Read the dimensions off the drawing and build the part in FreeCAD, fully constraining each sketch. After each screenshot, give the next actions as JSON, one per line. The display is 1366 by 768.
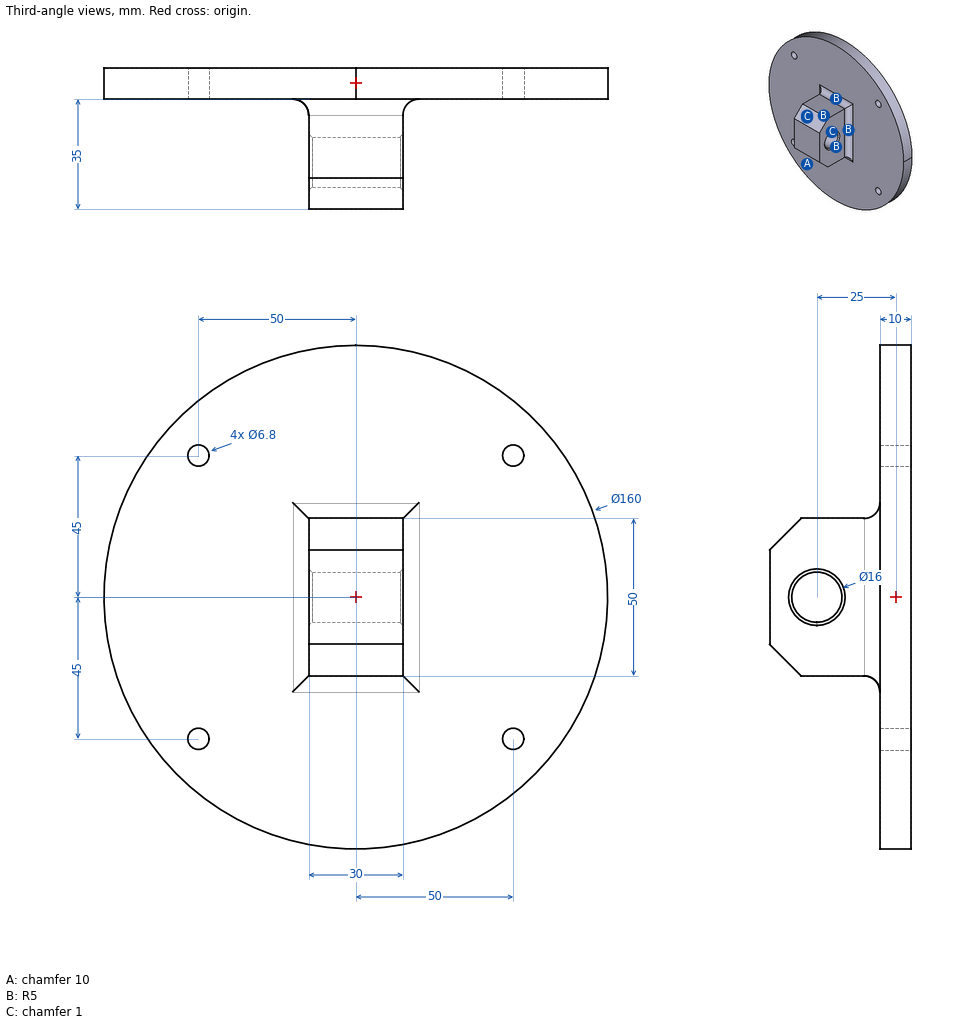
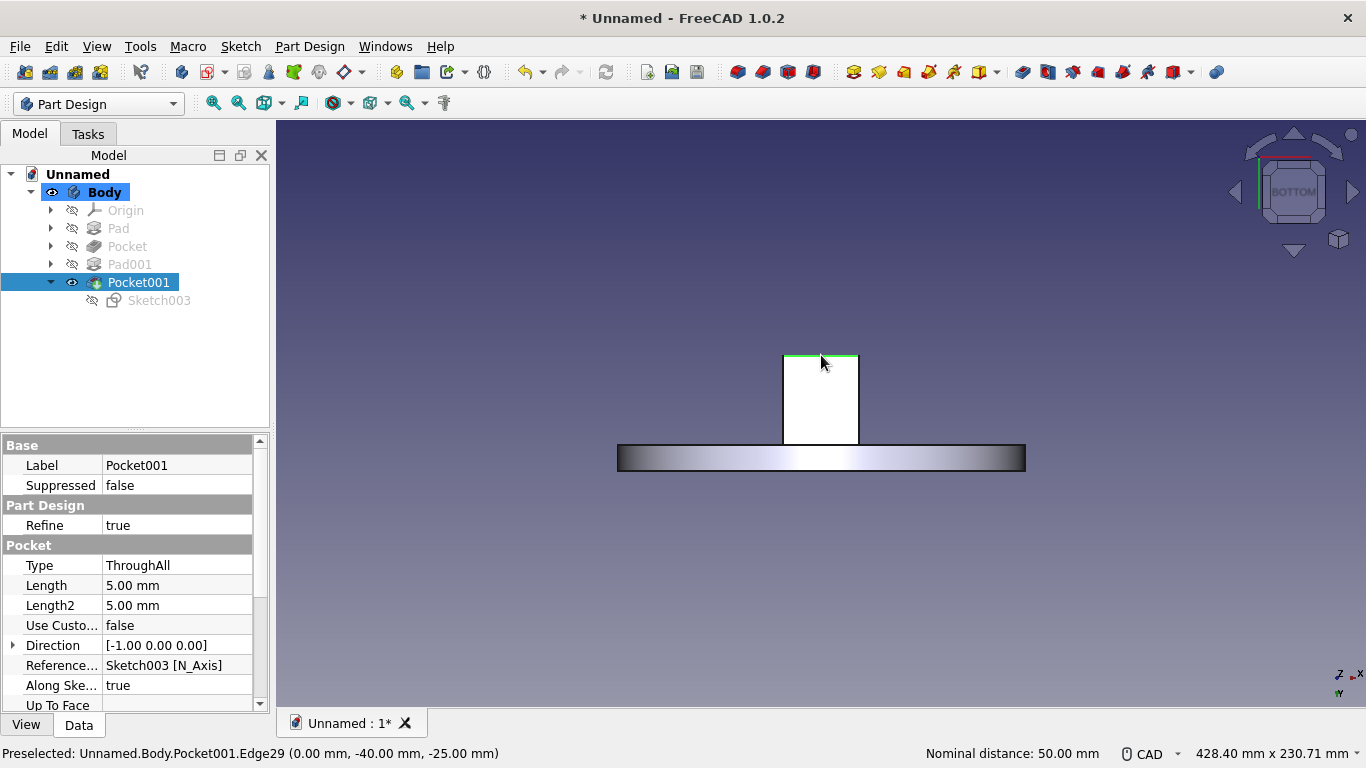
{"action": "left_click", "coordinate": [763, 72]}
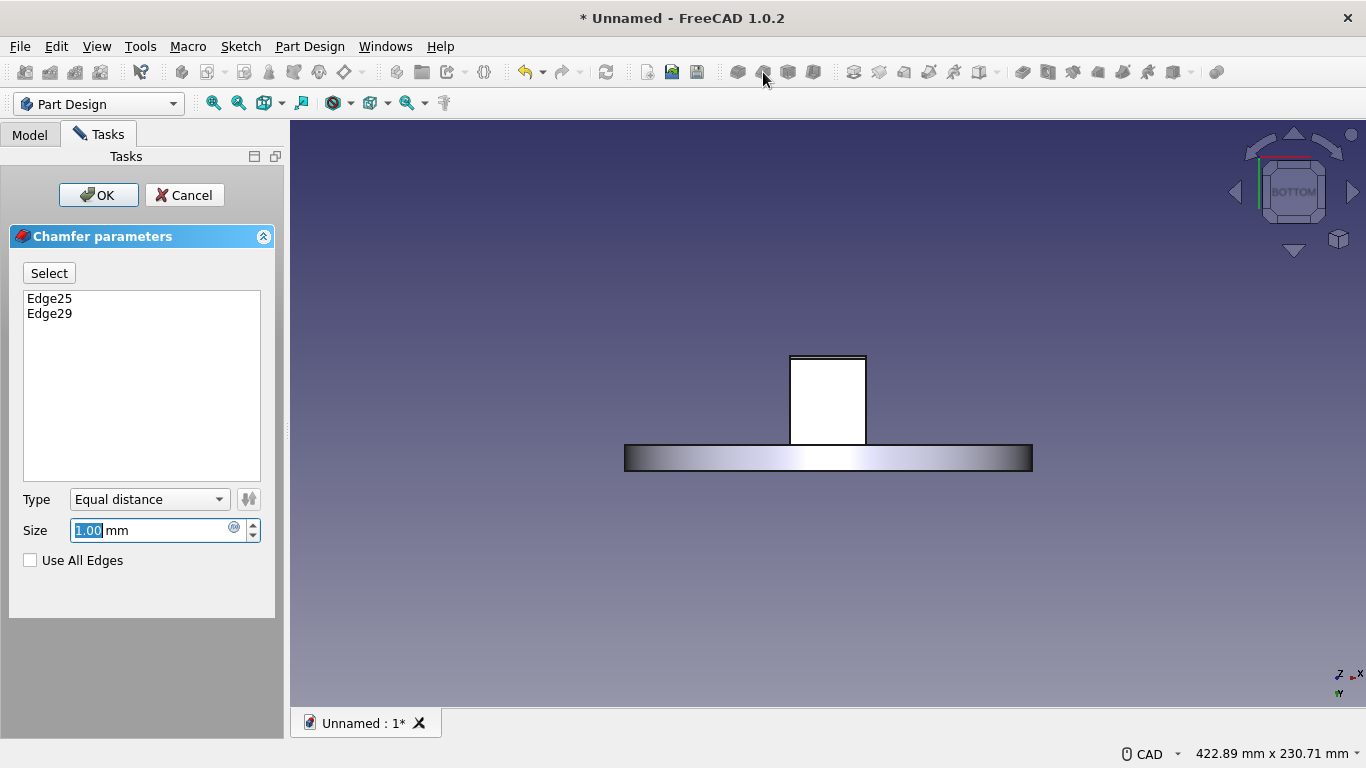
{"action": "type", "text": "10"}
{"action": "key", "text": "Tab"}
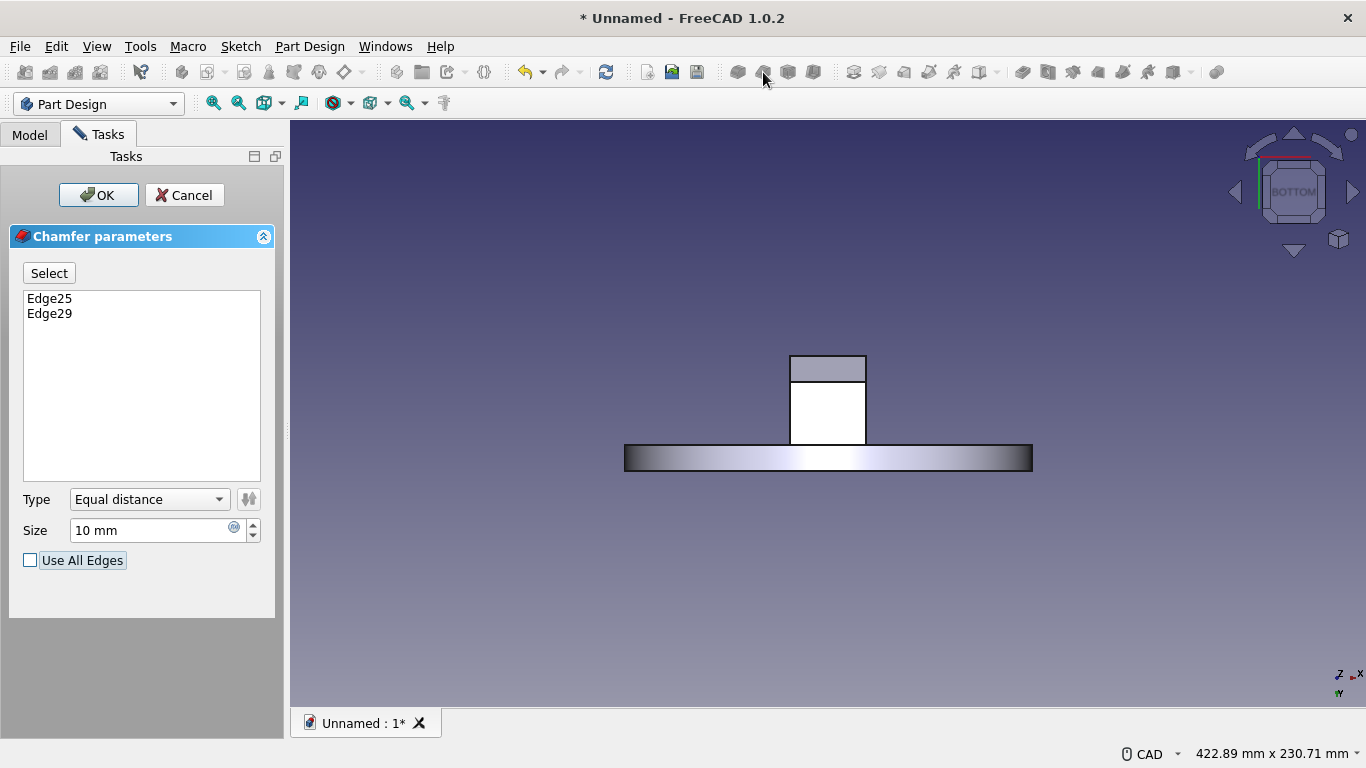
{"action": "left_click", "coordinate": [99, 195]}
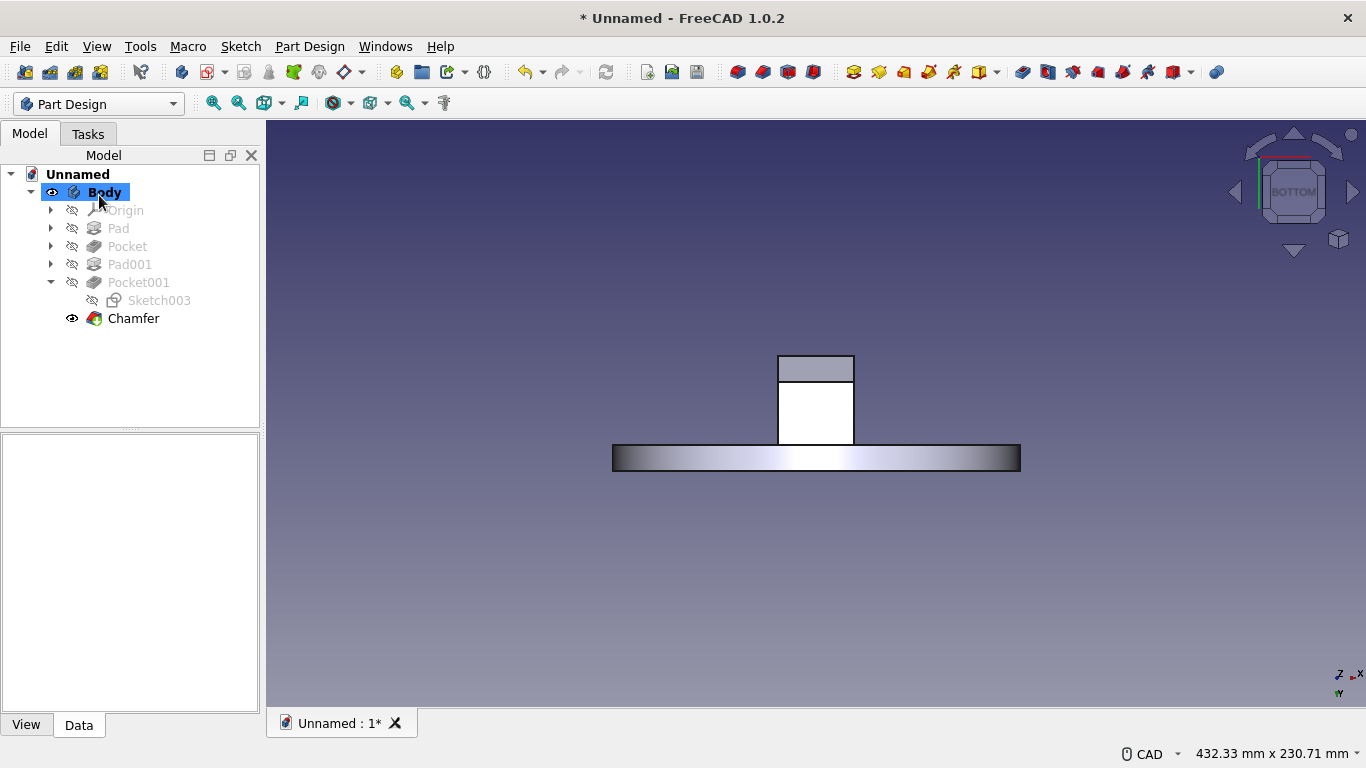
{"action": "key", "text": "v f"}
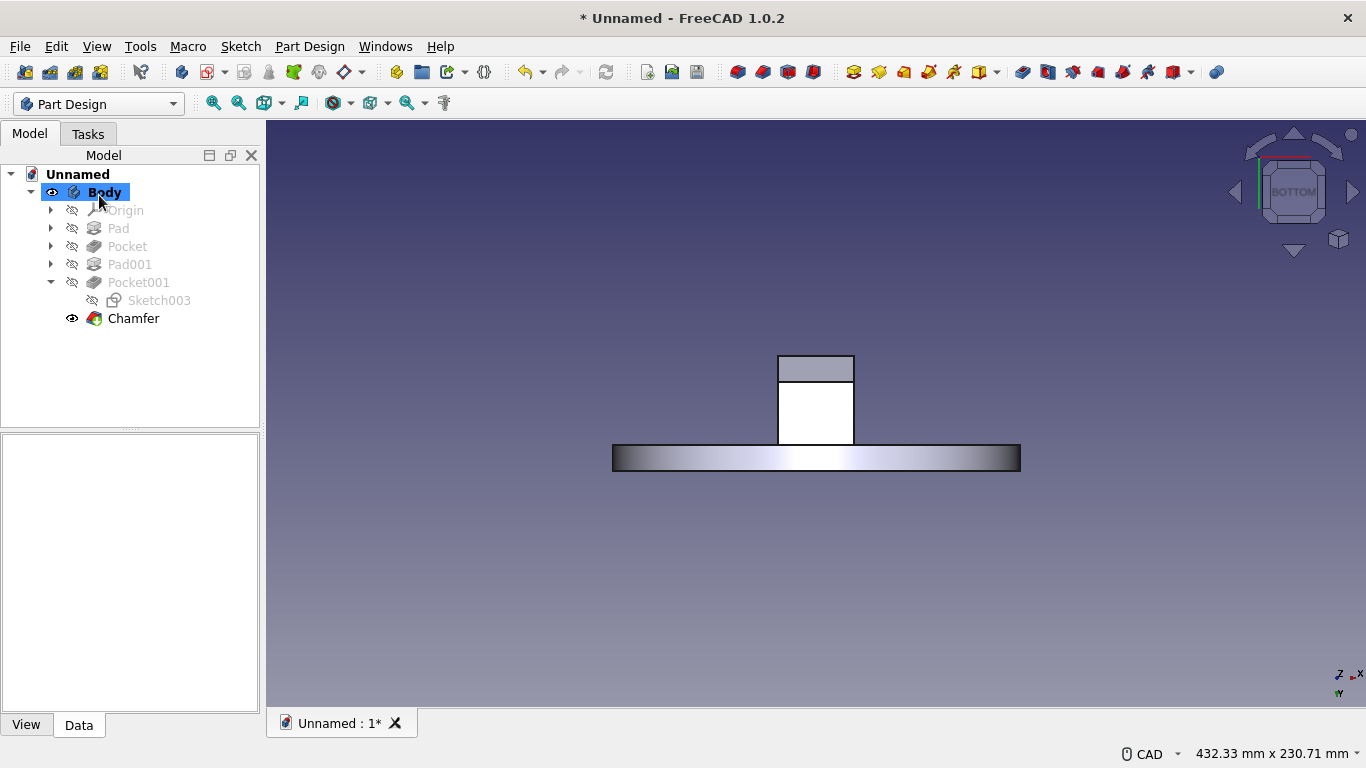
{"action": "key", "text": "0"}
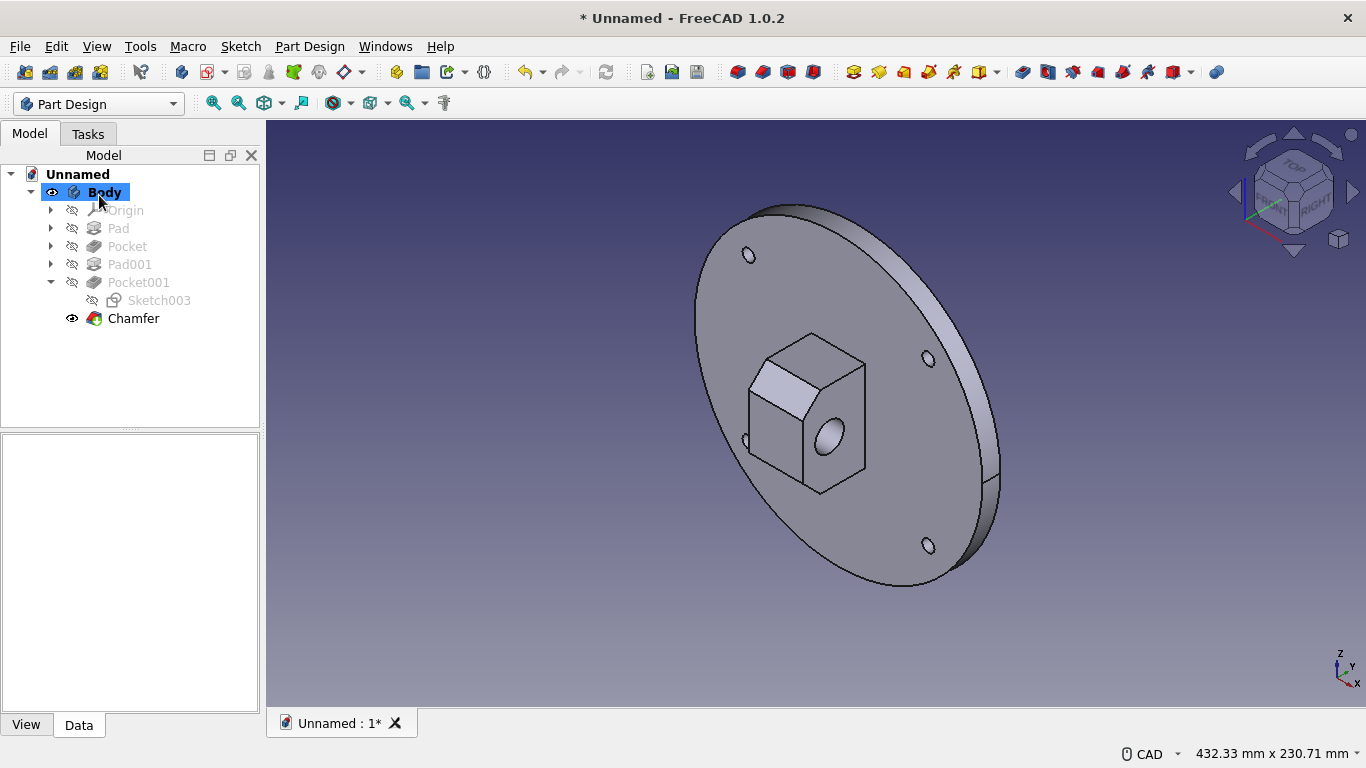
{"action": "key", "text": "2"}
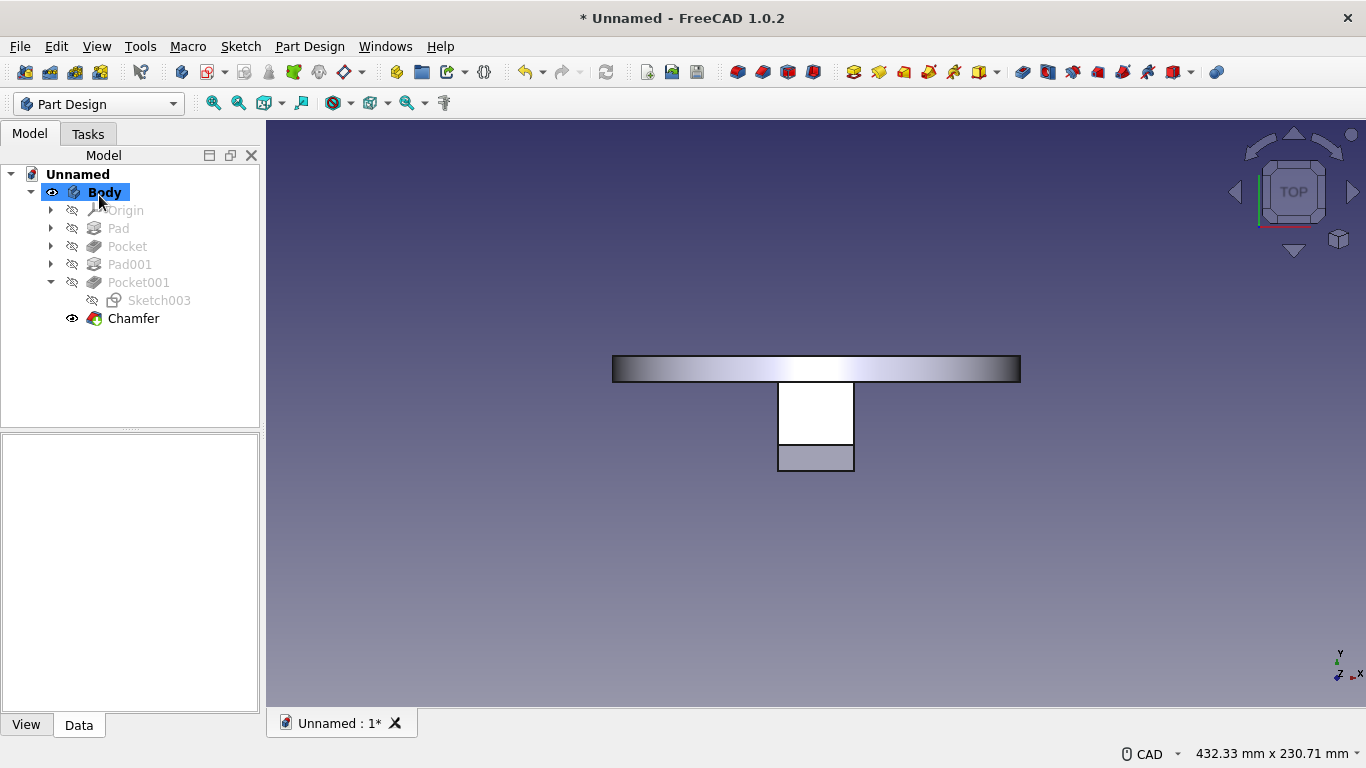
{"action": "key", "text": "v f"}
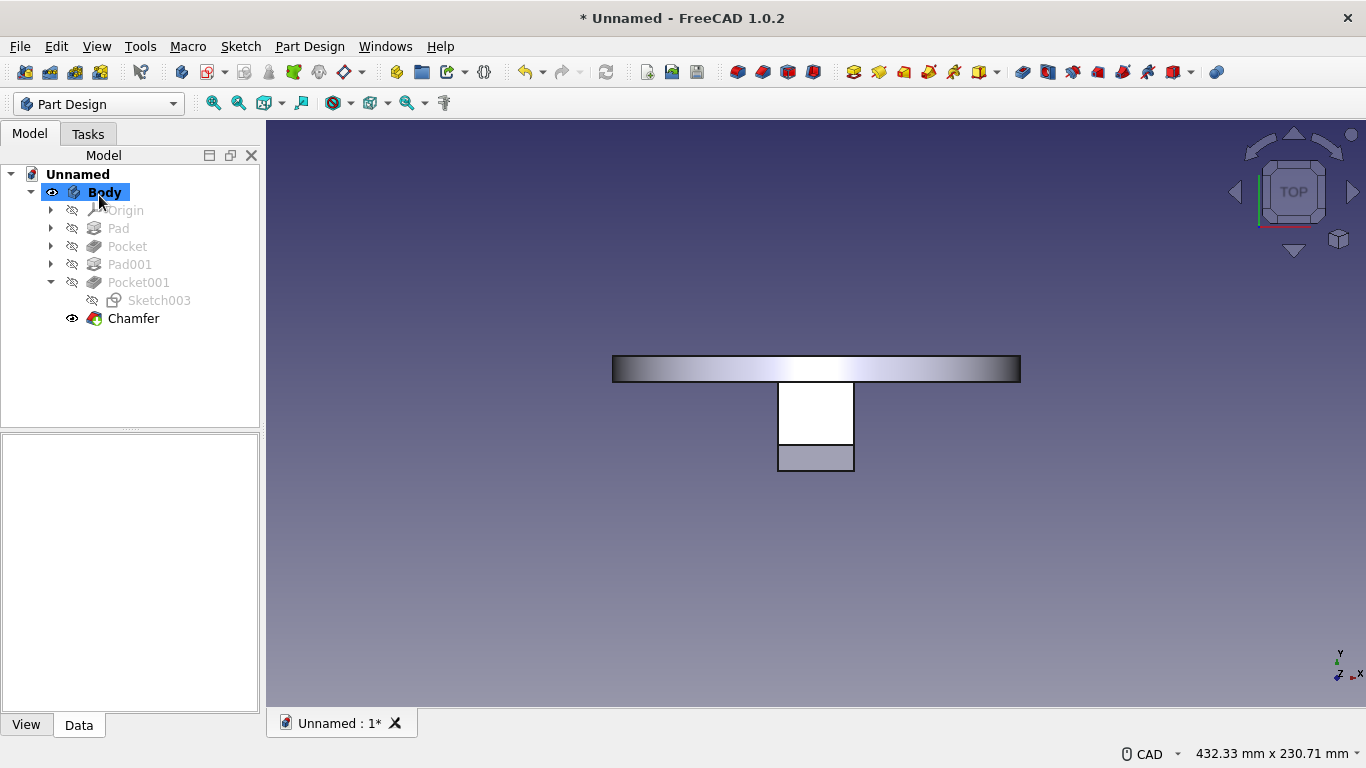
{"action": "key", "text": "1"}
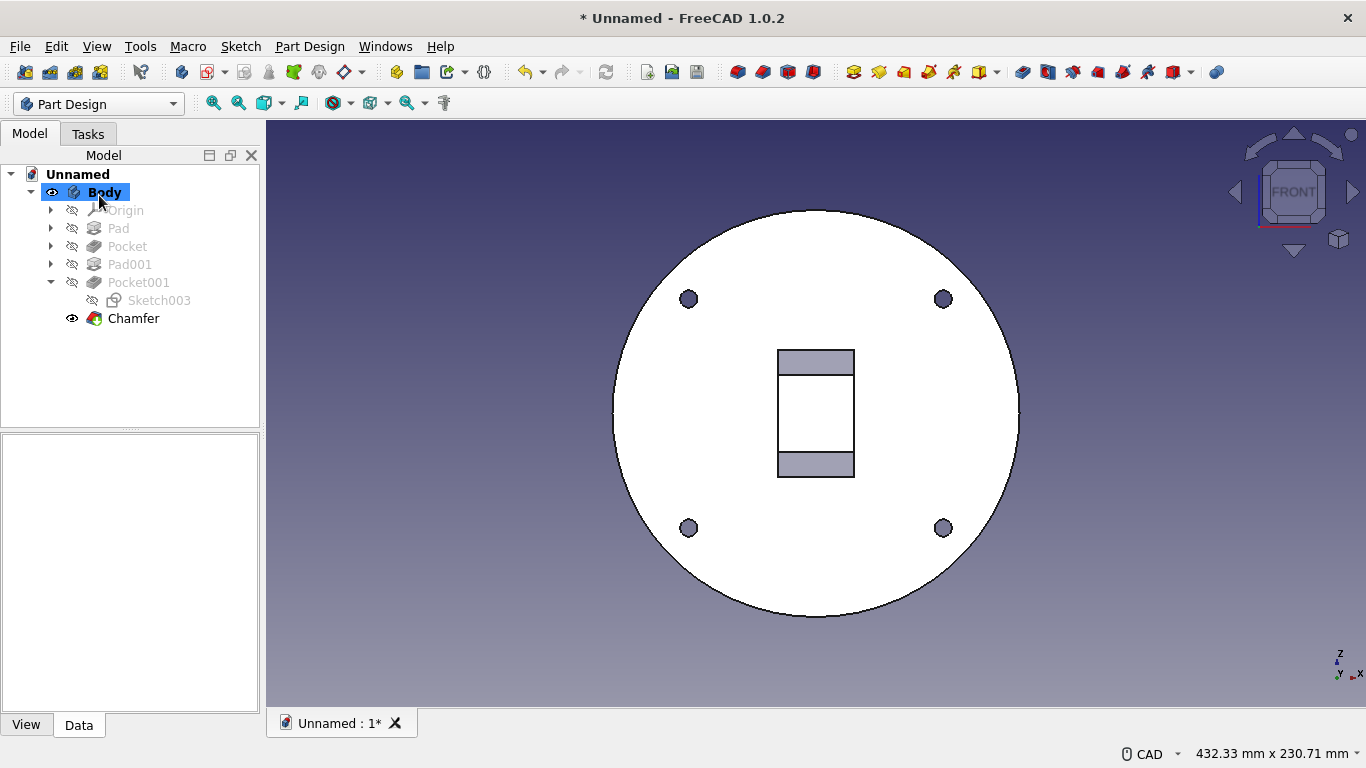
{"action": "key", "text": "3"}